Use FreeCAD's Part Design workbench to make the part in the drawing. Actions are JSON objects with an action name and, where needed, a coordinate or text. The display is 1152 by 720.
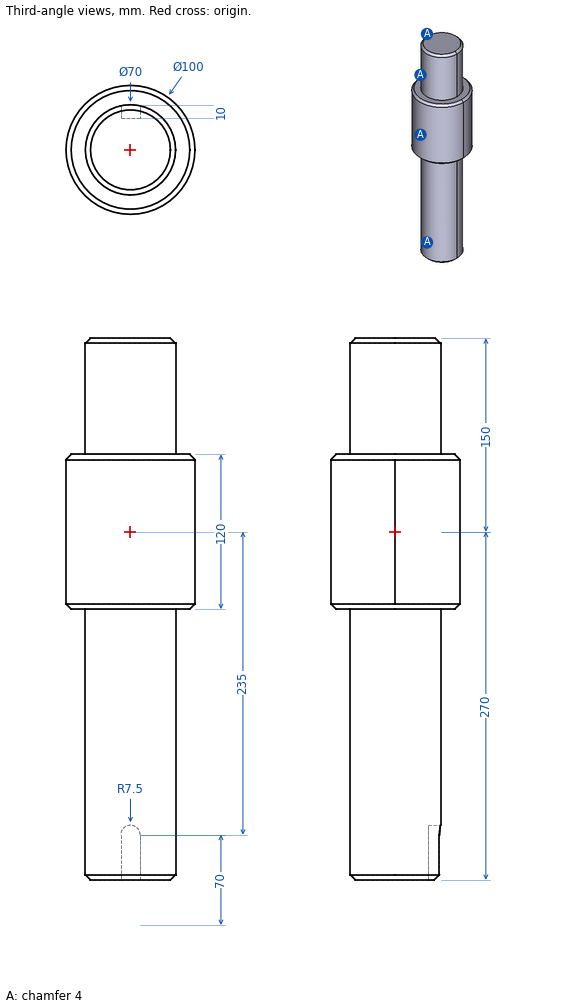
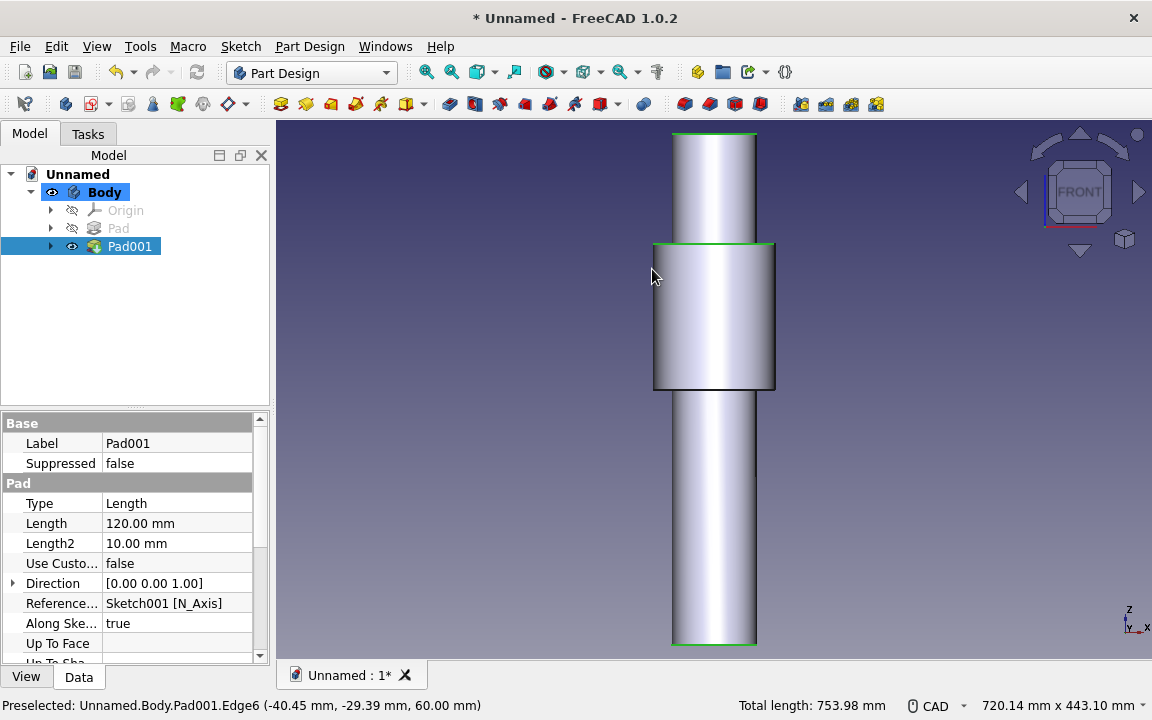
{"action": "left_click", "coordinate": [665, 389], "text": "ctrl"}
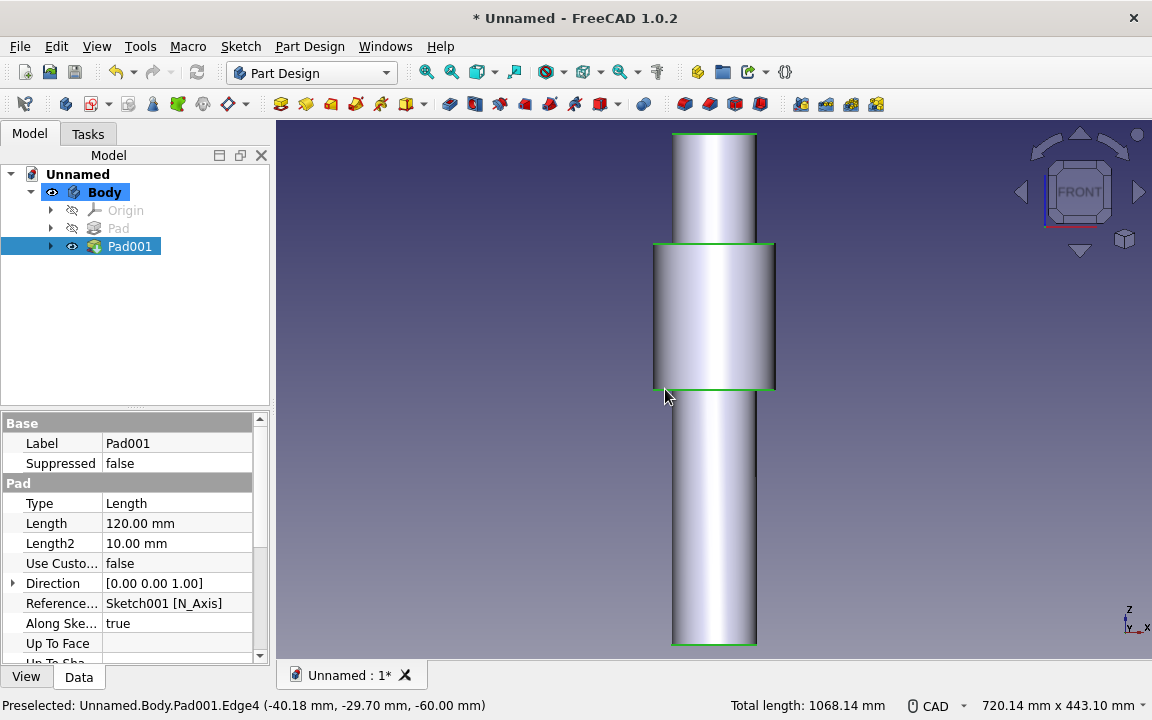
{"action": "left_click", "coordinate": [710, 104]}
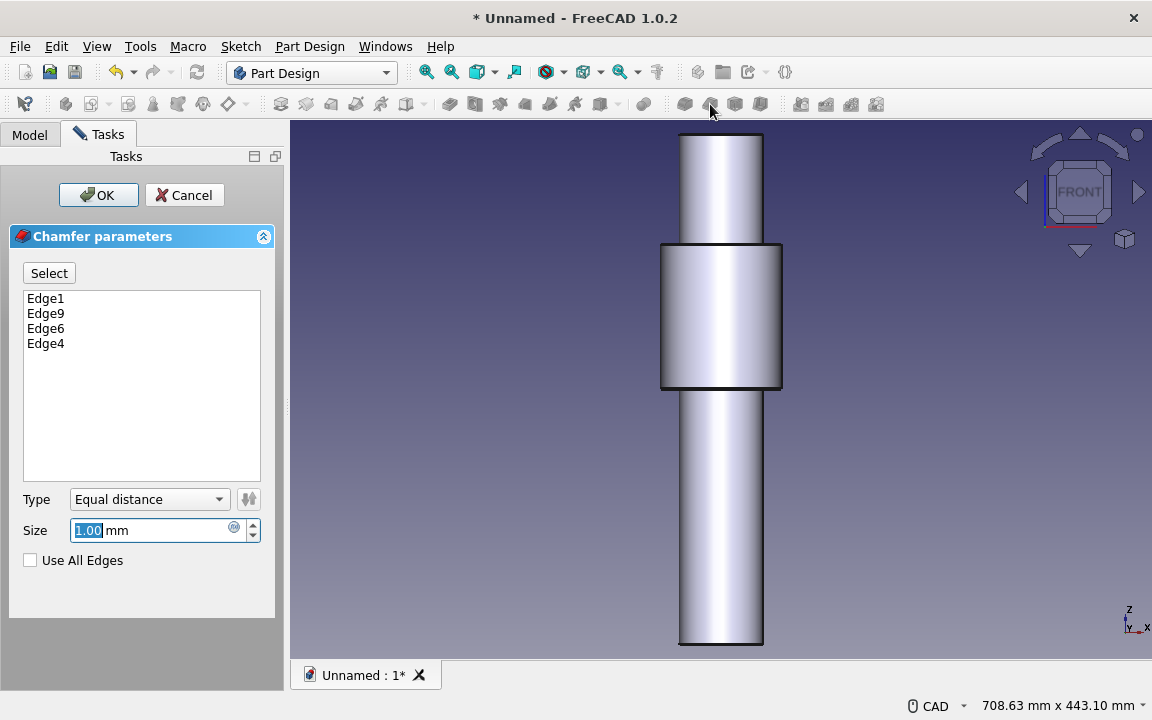
{"action": "type", "text": "4"}
{"action": "key", "text": "Tab"}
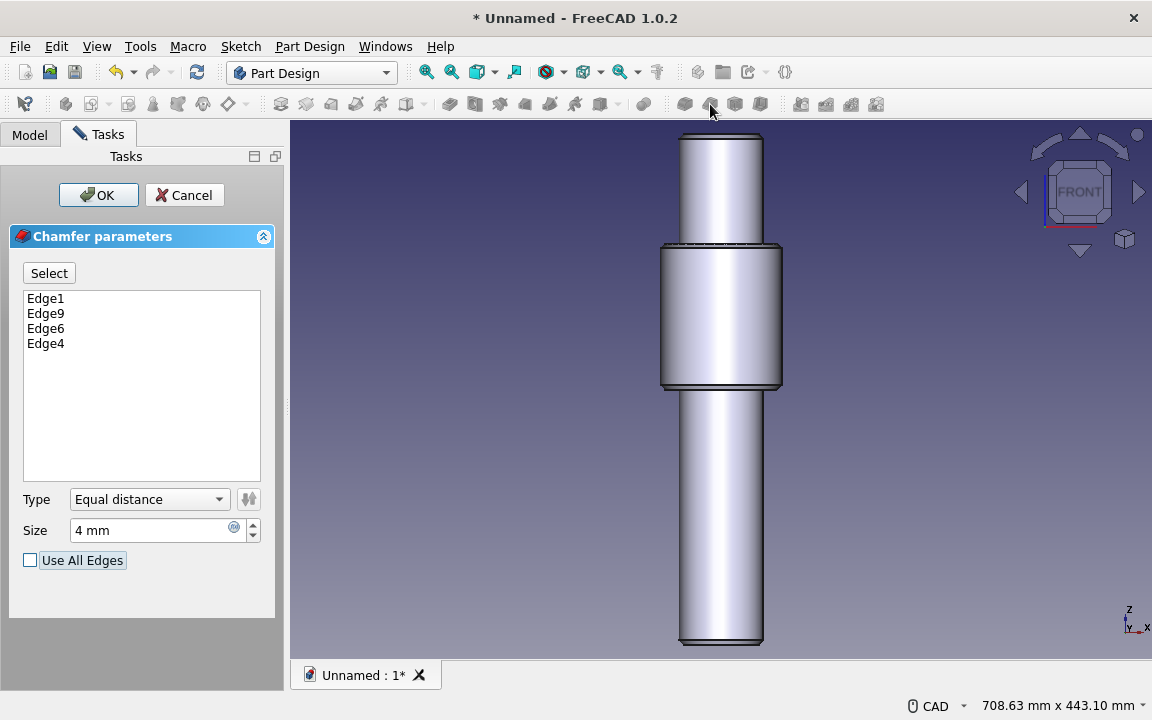
{"action": "left_click", "coordinate": [99, 195]}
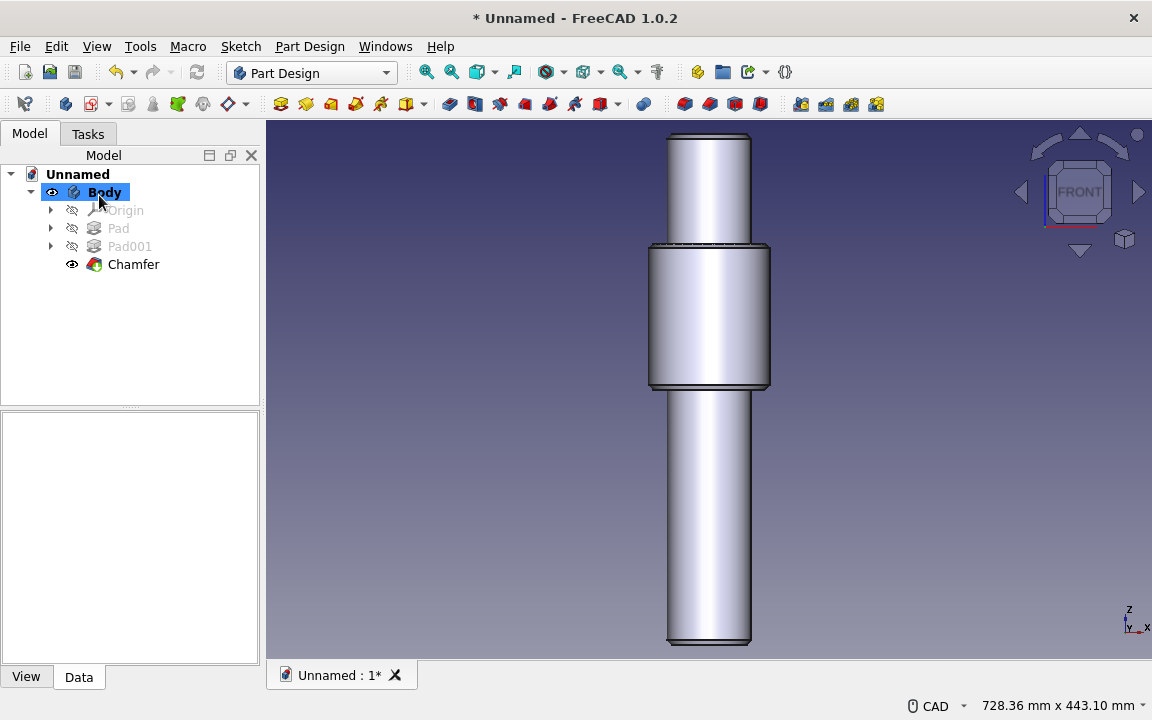
{"action": "left_click", "coordinate": [51, 210]}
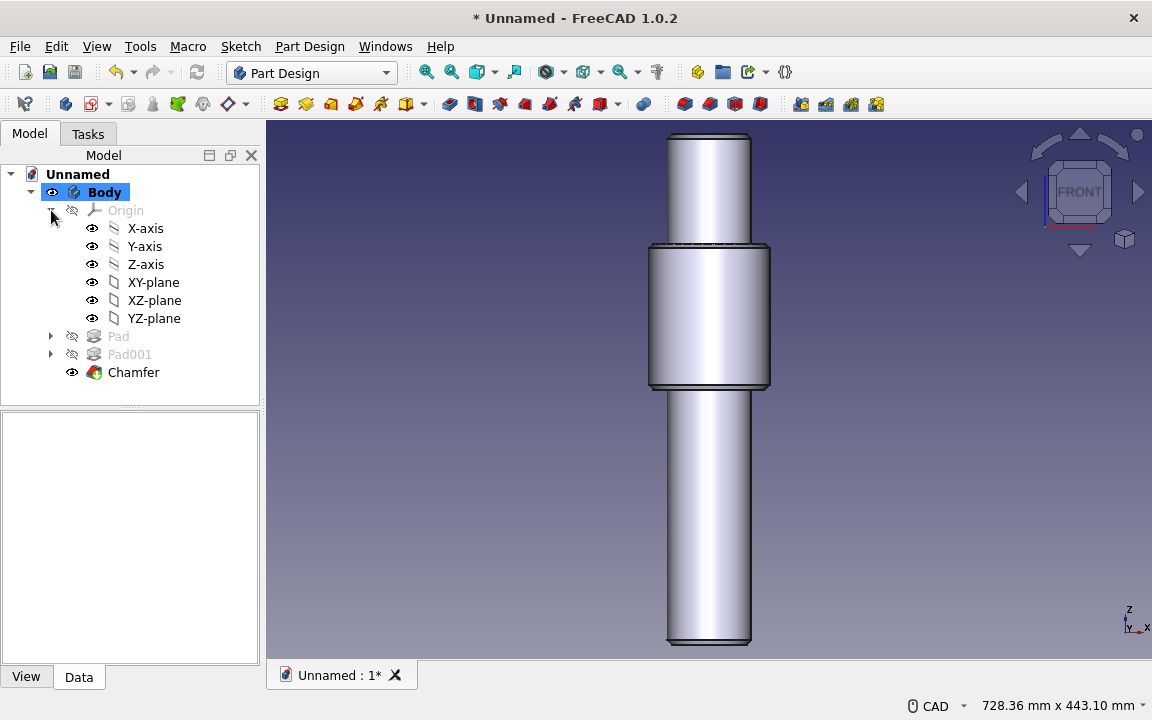
{"action": "left_click", "coordinate": [137, 300]}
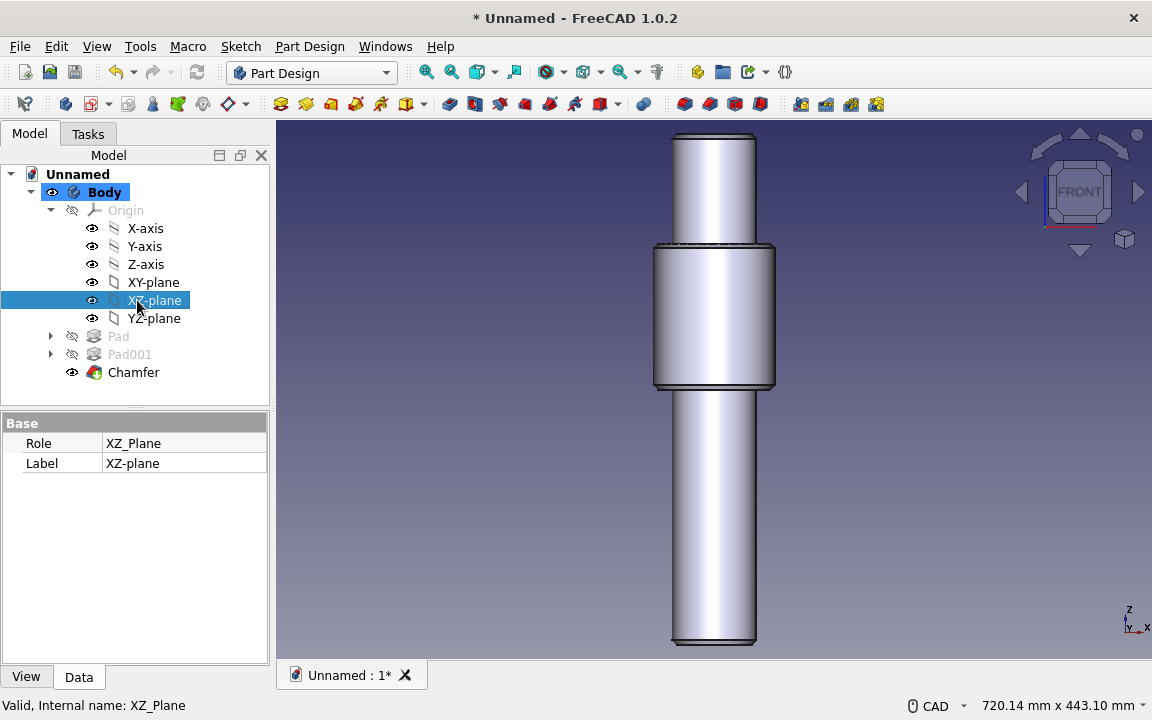
{"action": "left_click", "coordinate": [228, 104]}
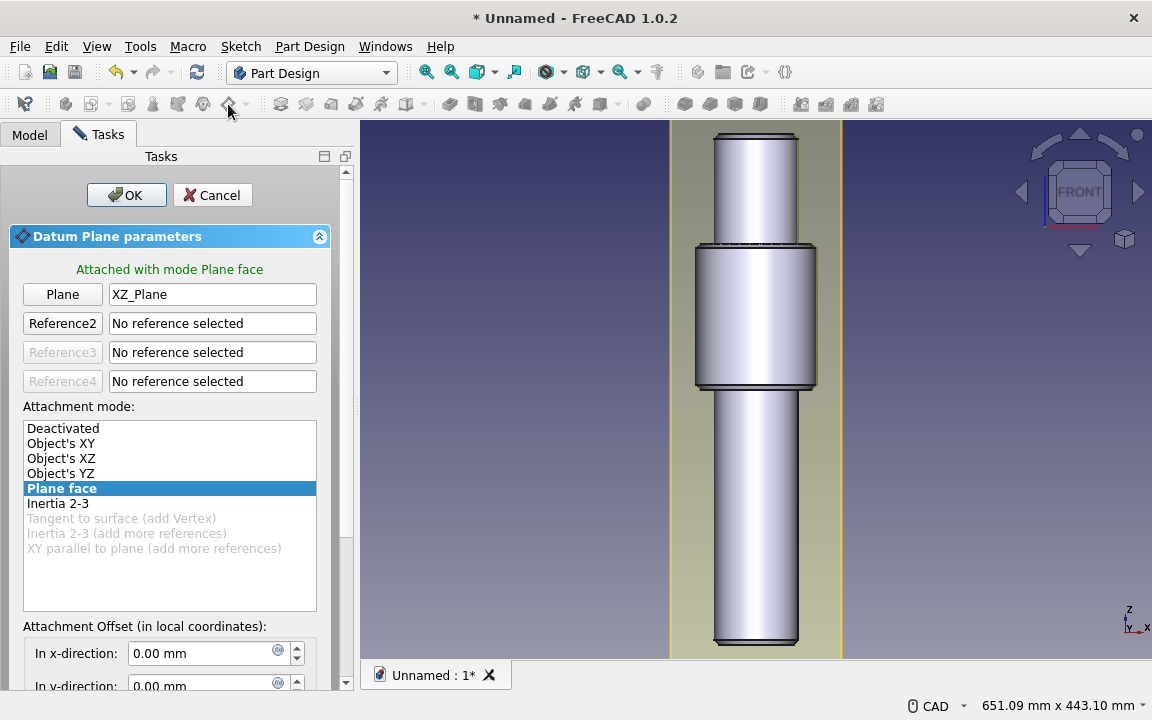
{"action": "scroll", "coordinate": [346, 428], "scroll_direction": "down", "scroll_amount": 2}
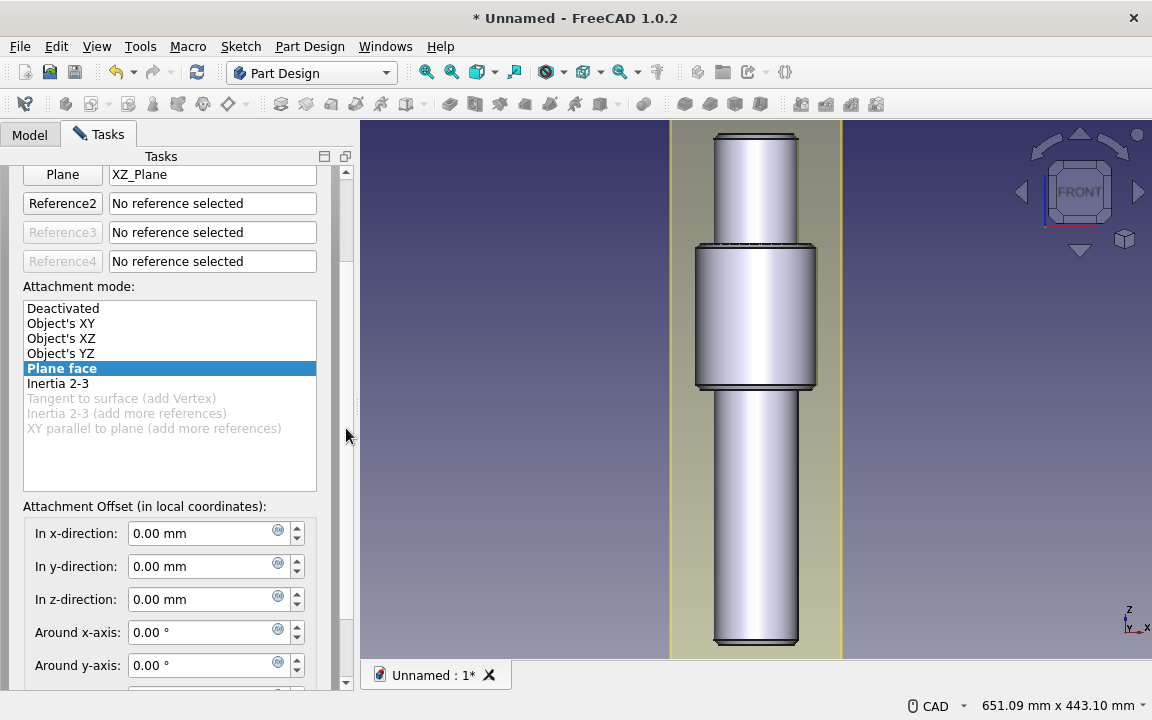
{"action": "triple_click", "coordinate": [210, 600]}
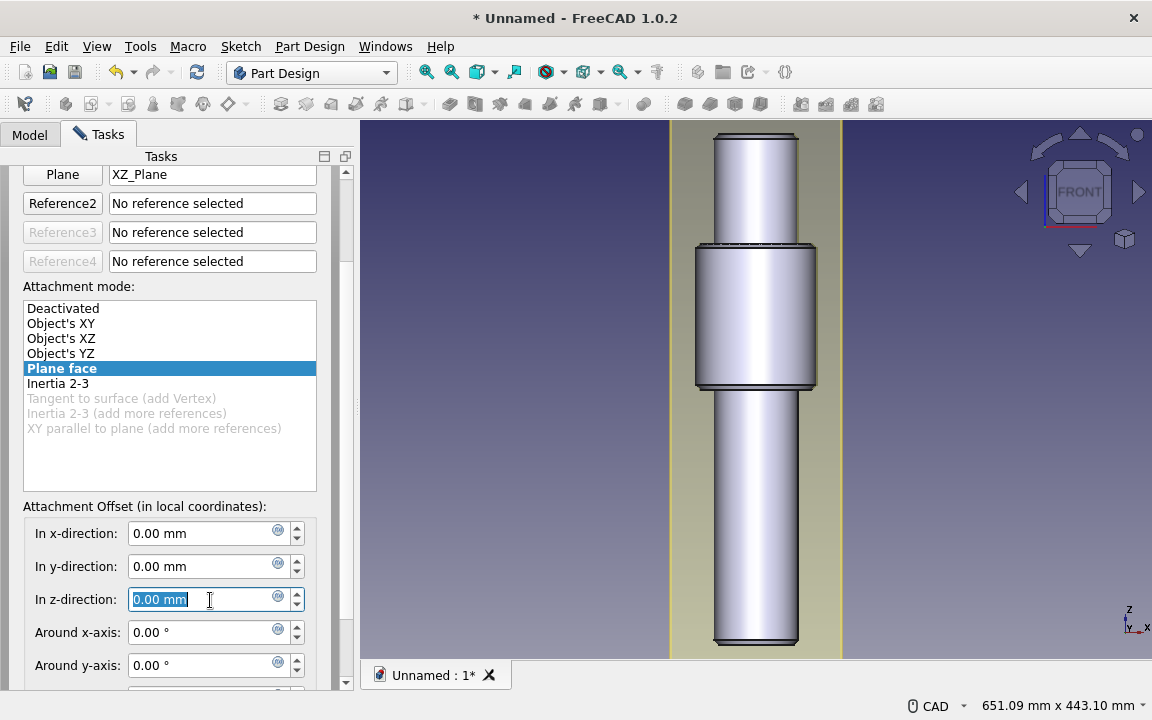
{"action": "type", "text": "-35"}
{"action": "key", "text": "Tab"}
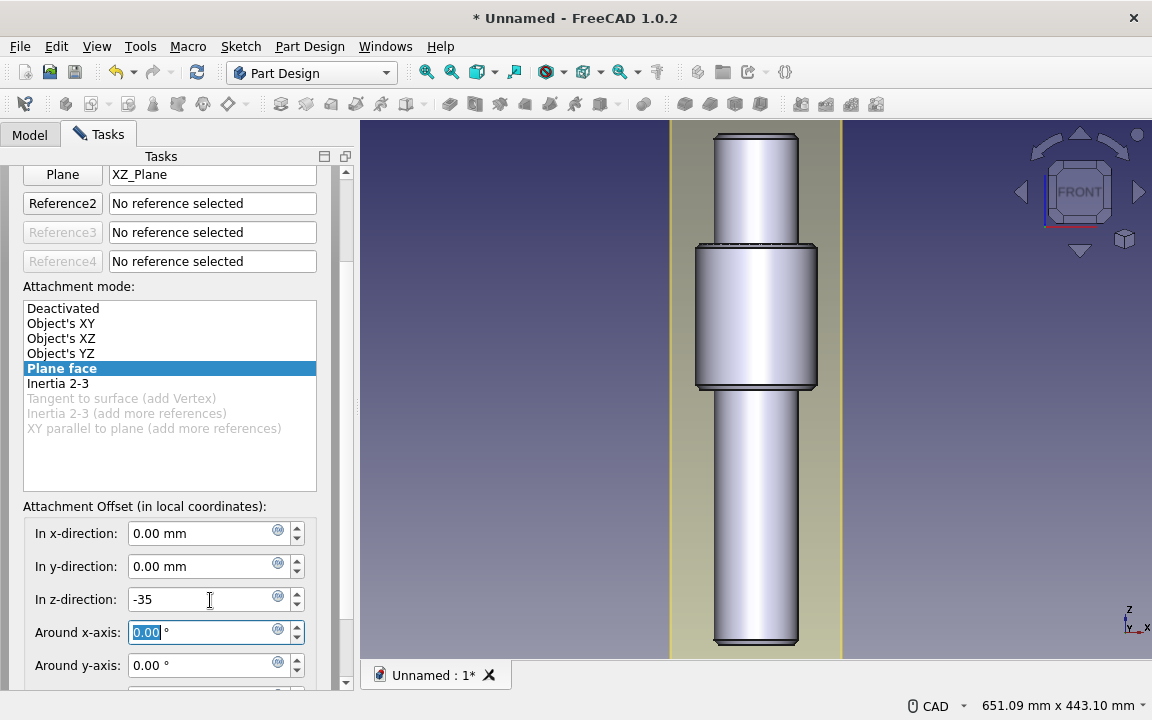
{"action": "scroll", "coordinate": [346, 428], "scroll_direction": "up", "scroll_amount": 3}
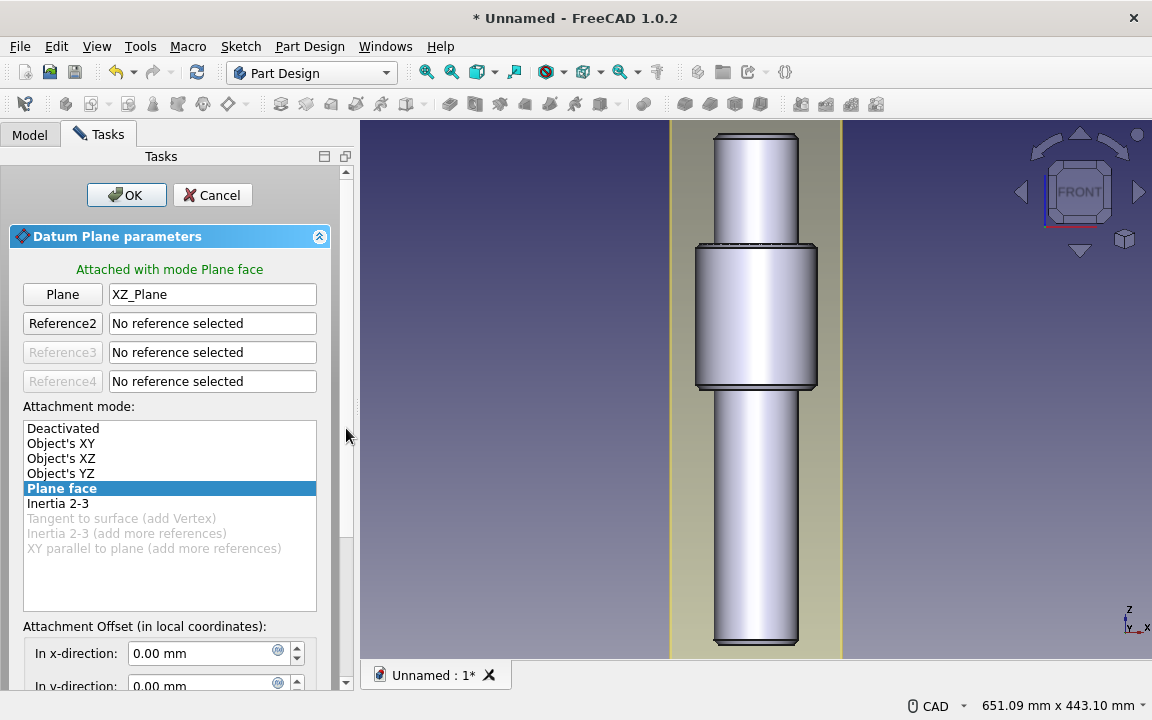
{"action": "left_click", "coordinate": [127, 195]}